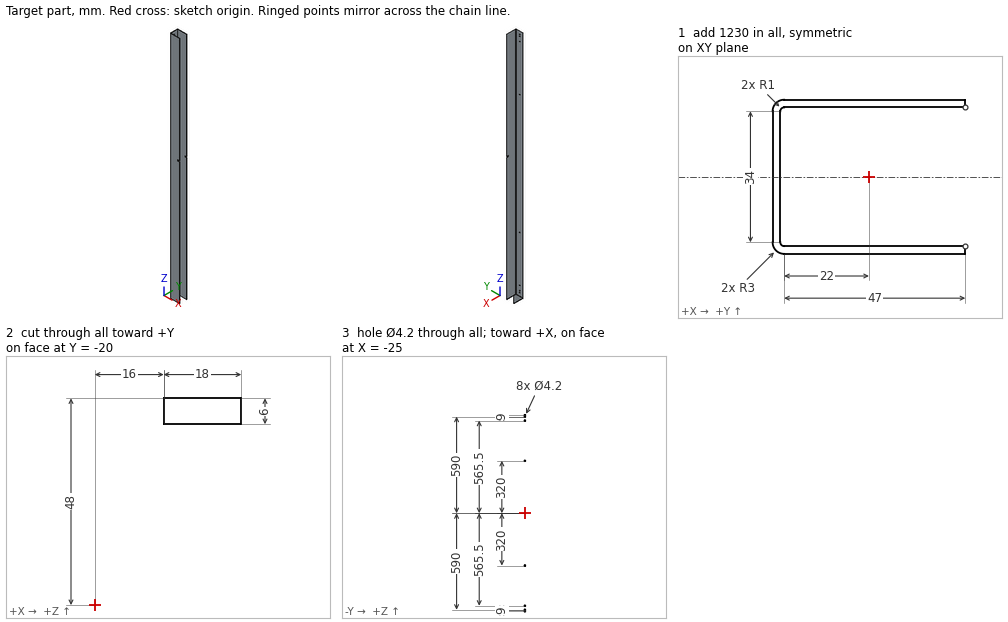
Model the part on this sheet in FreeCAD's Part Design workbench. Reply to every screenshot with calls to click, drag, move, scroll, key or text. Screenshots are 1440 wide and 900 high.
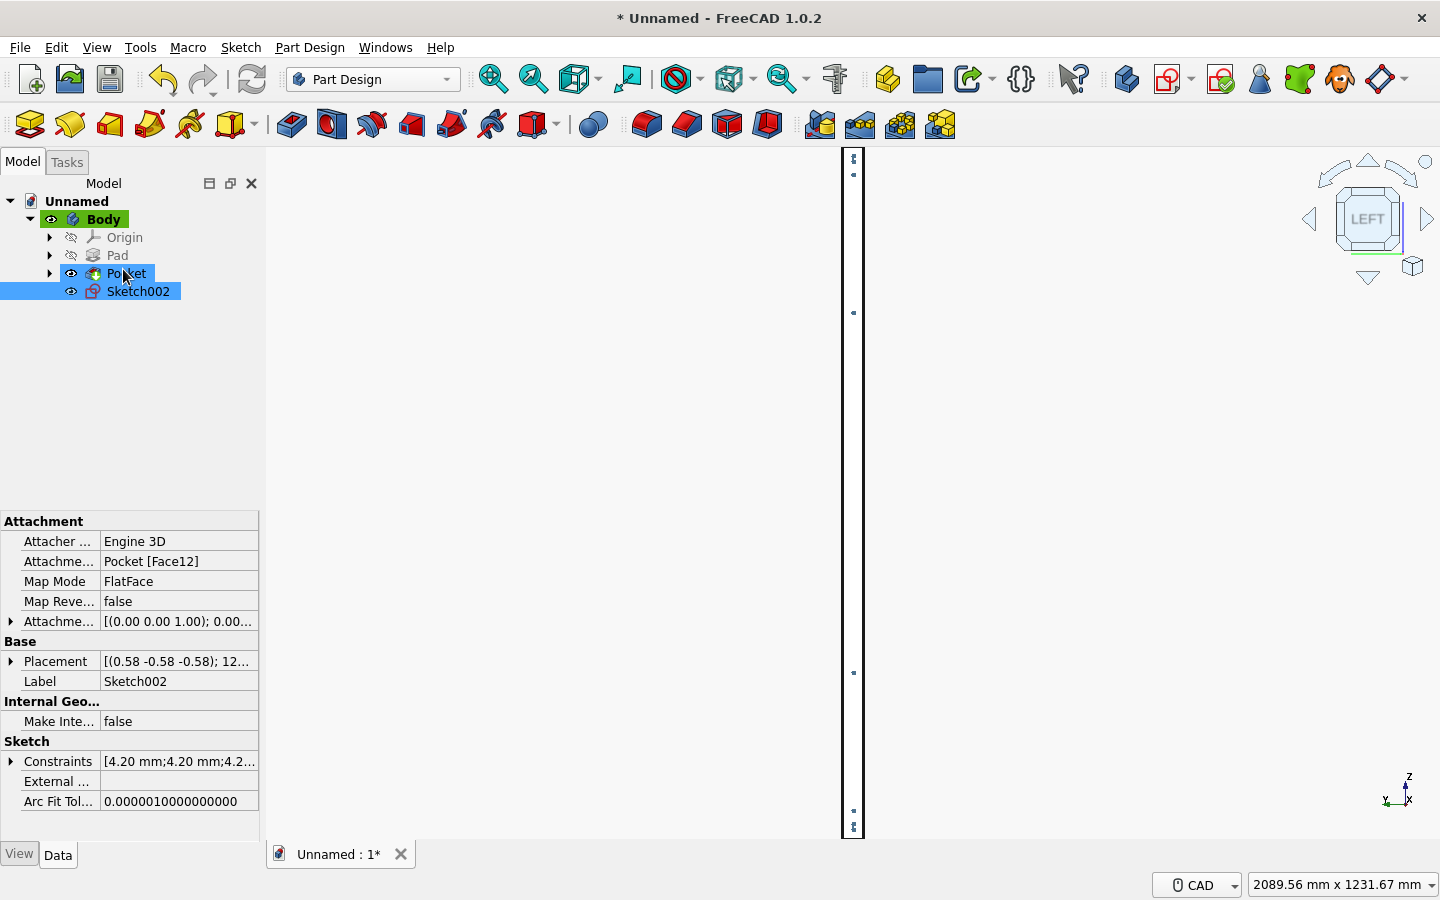
click(332, 124)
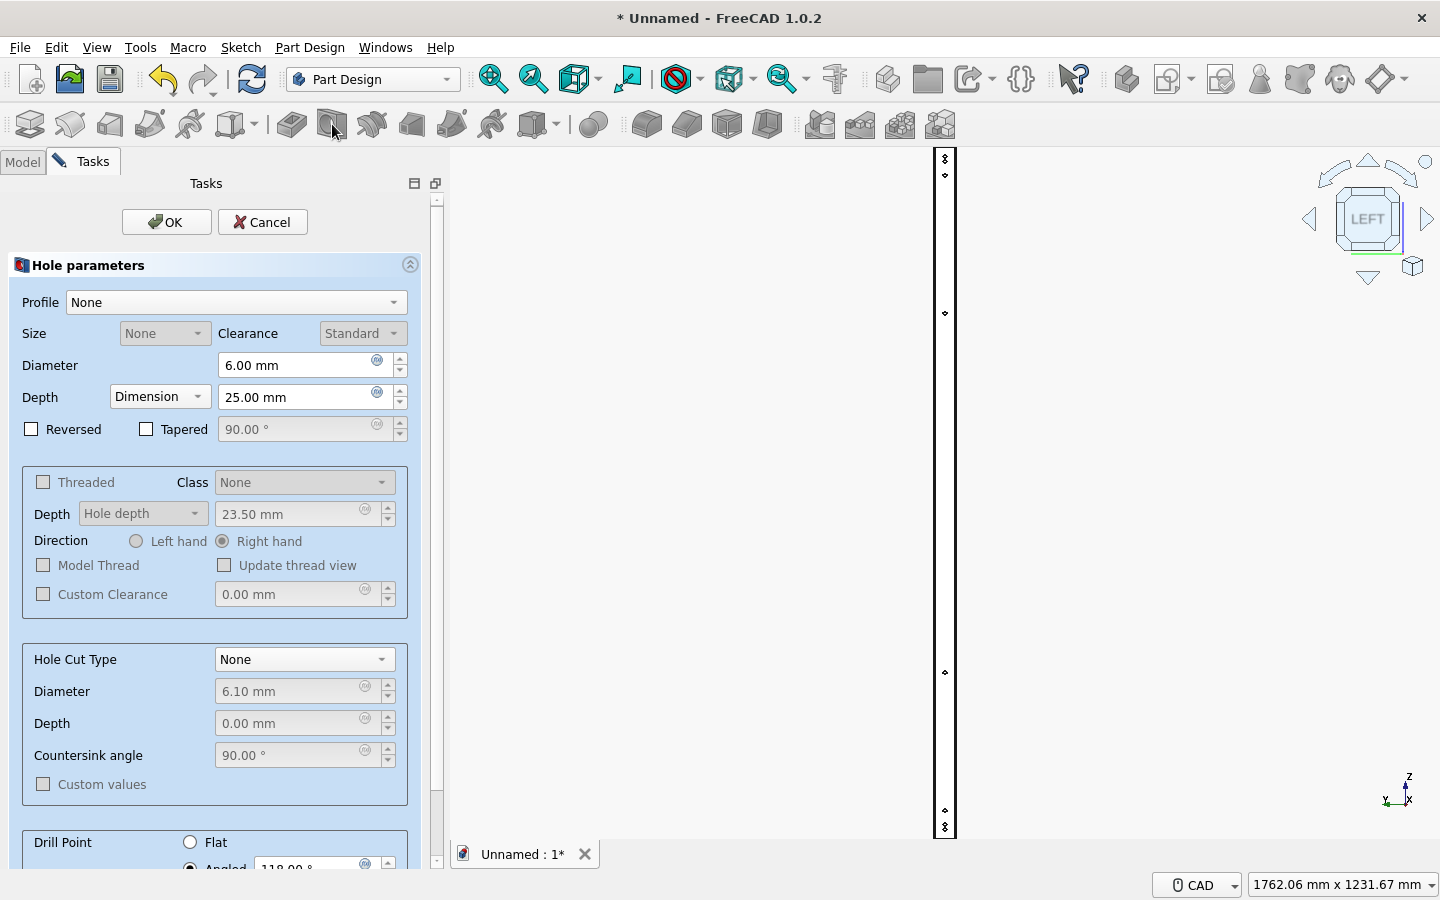
triple_click(305, 365)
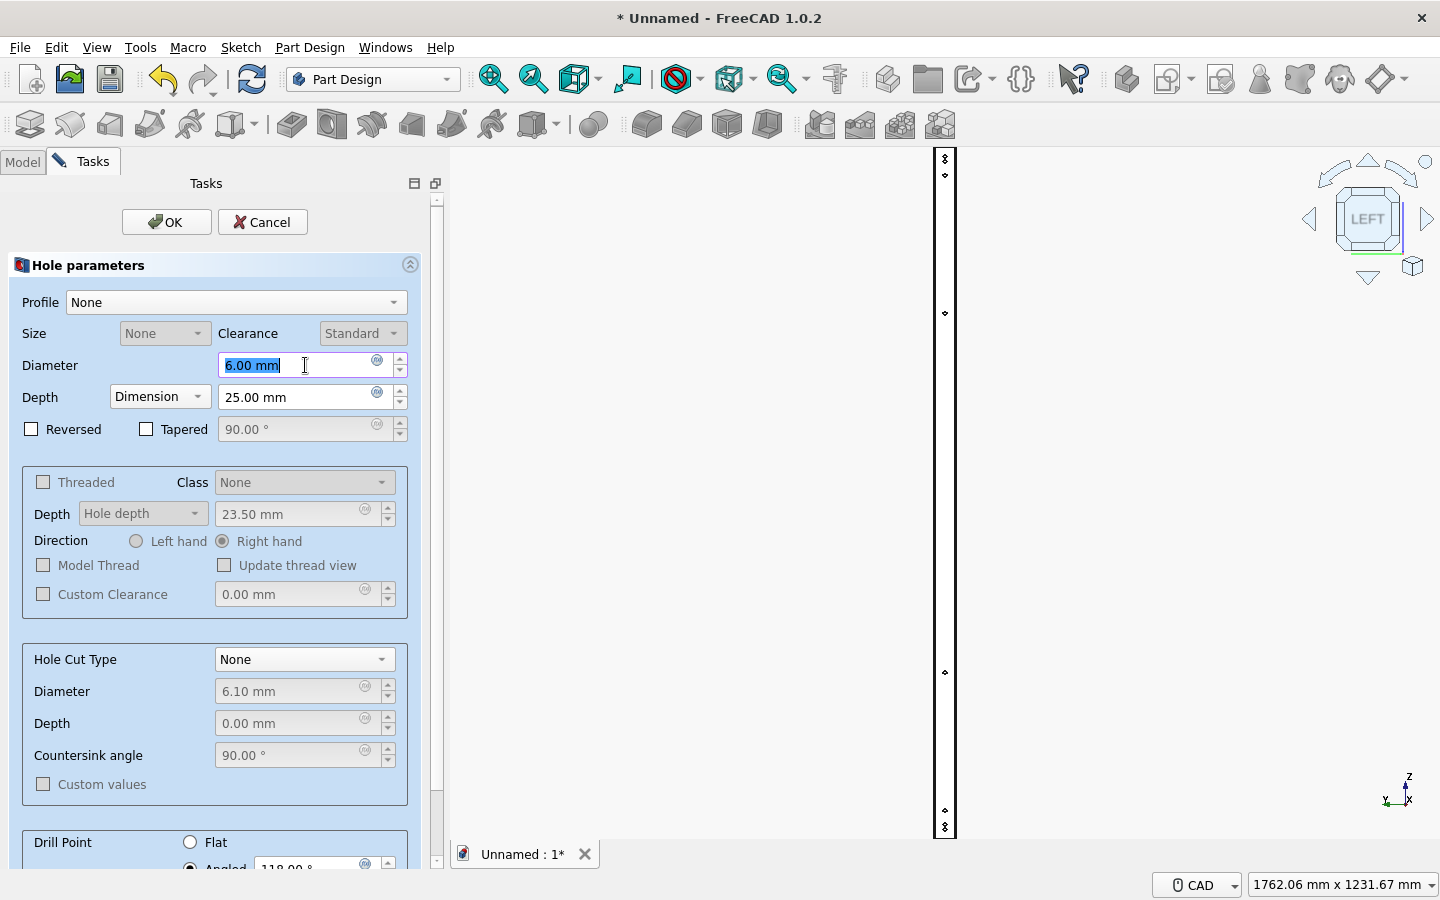
text(4.2)
key(Tab)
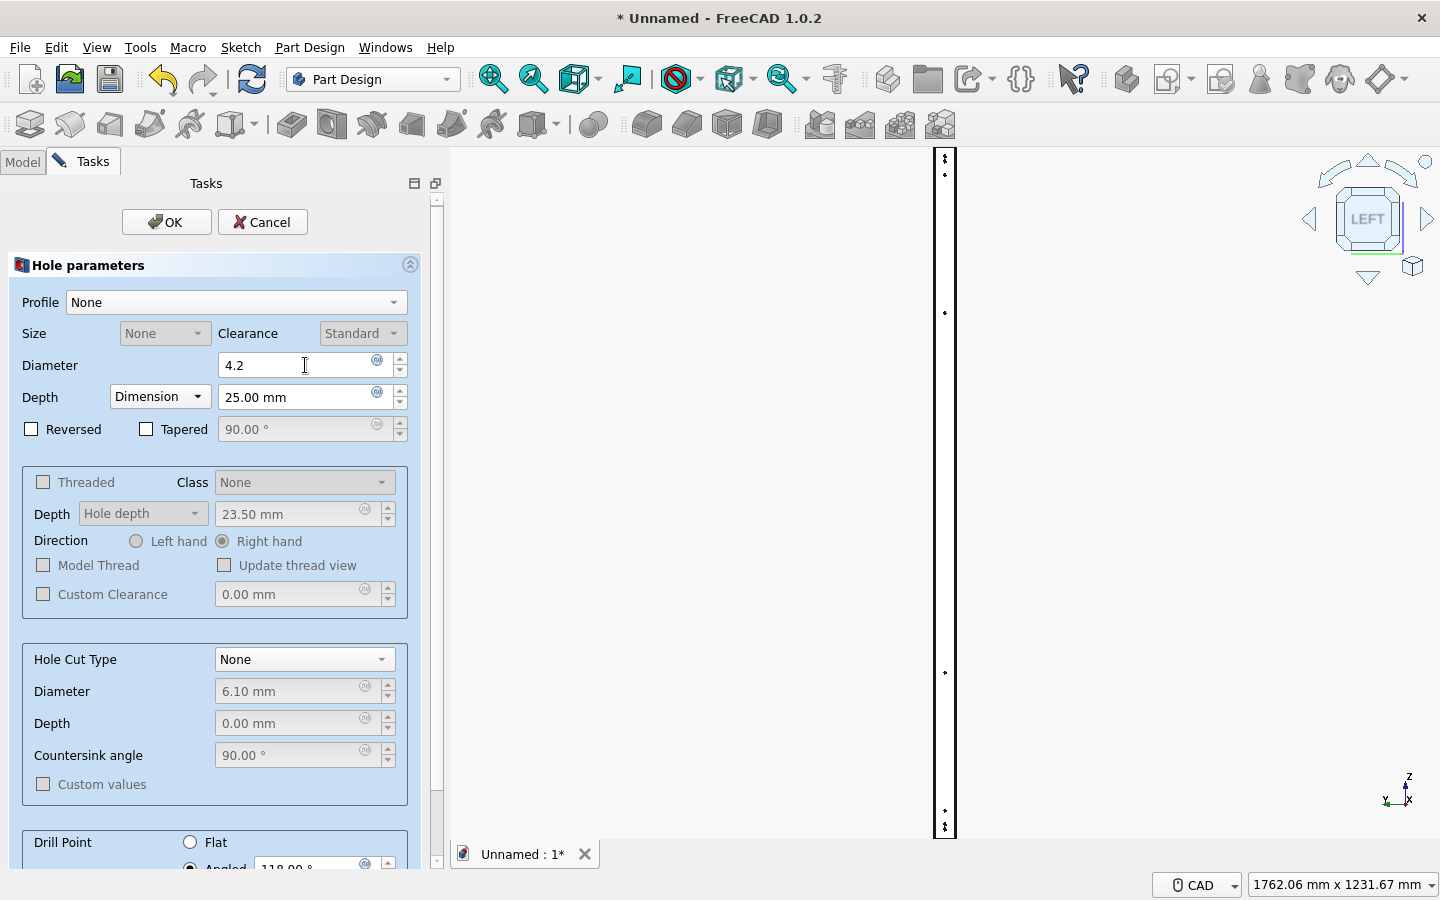
click(161, 396)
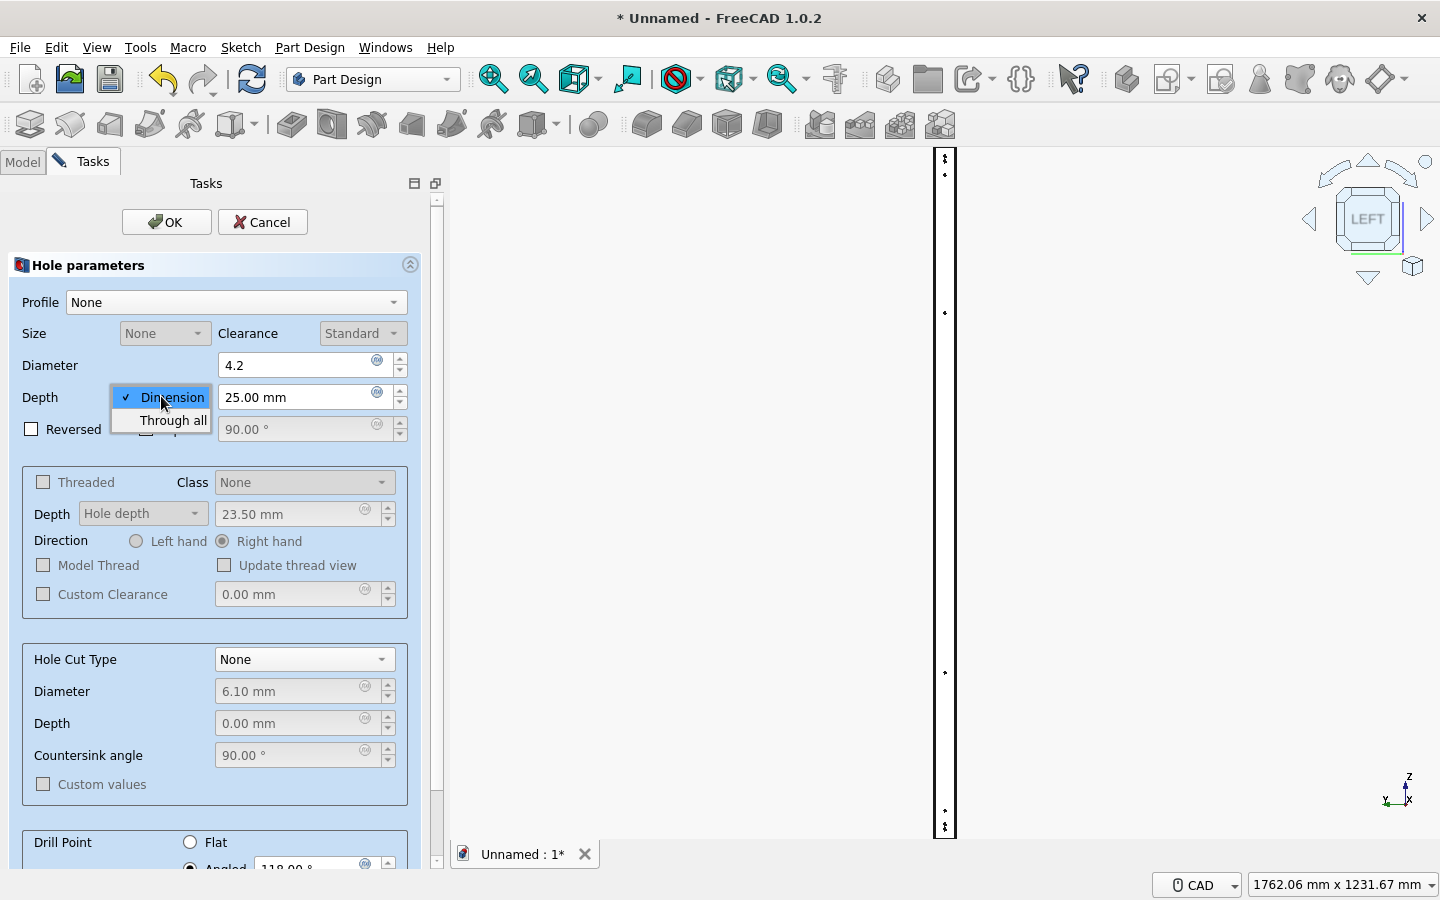
click(160, 420)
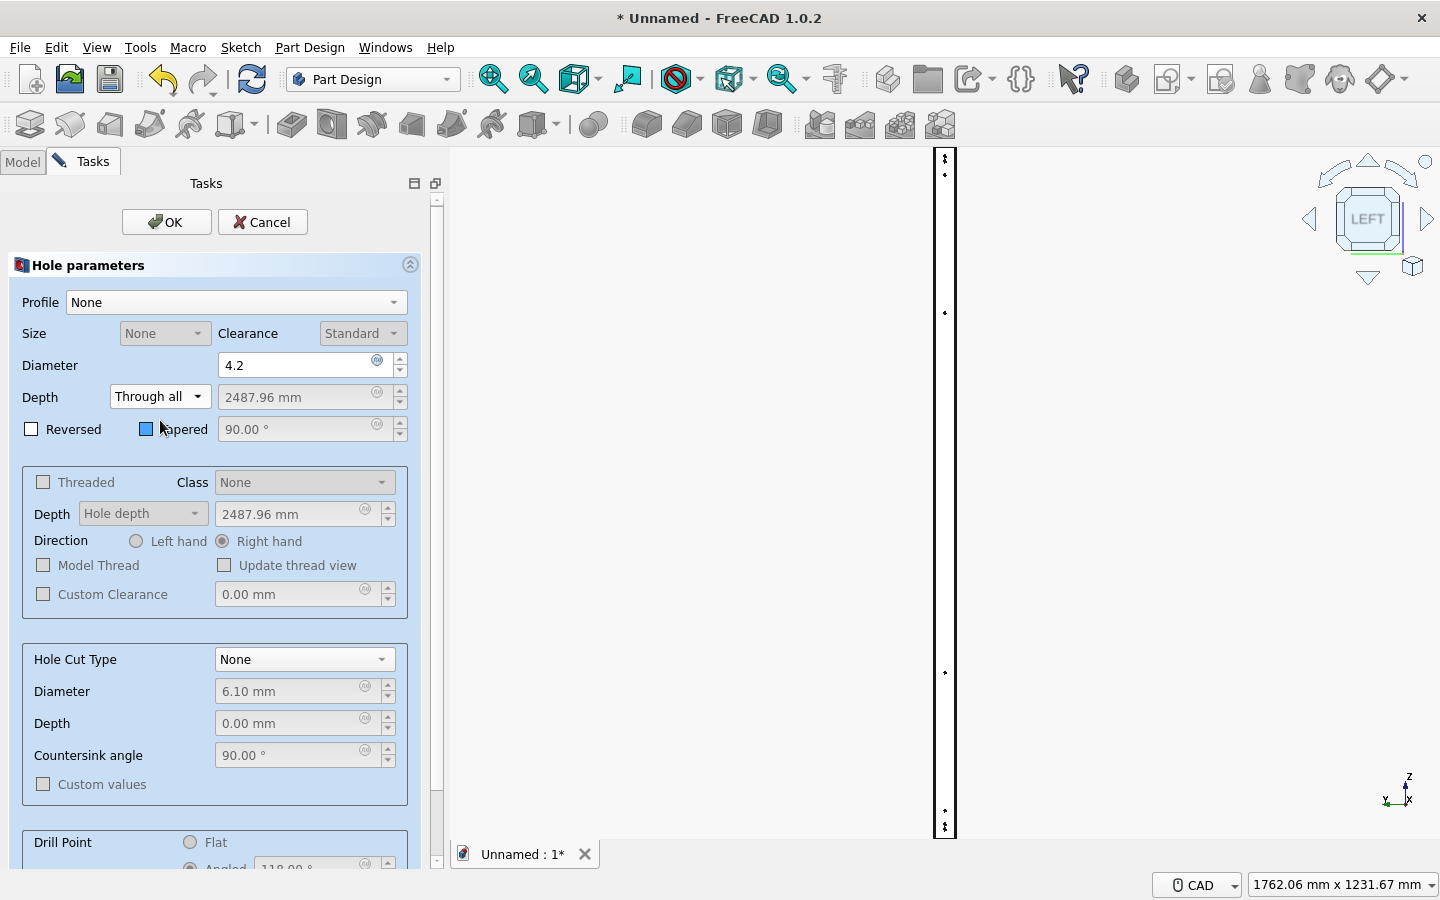
click(167, 222)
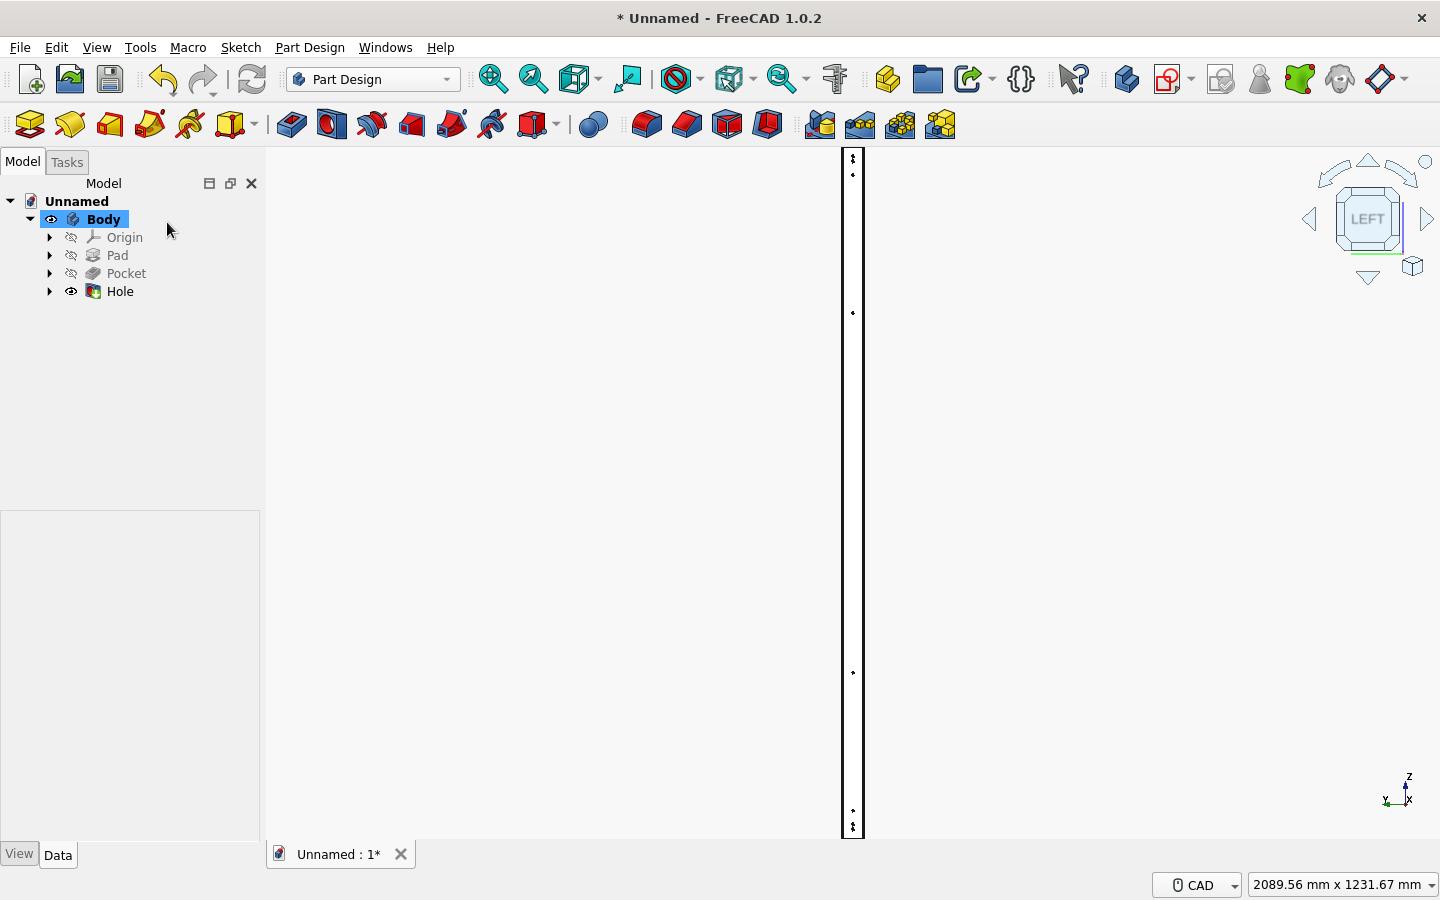
key(0)